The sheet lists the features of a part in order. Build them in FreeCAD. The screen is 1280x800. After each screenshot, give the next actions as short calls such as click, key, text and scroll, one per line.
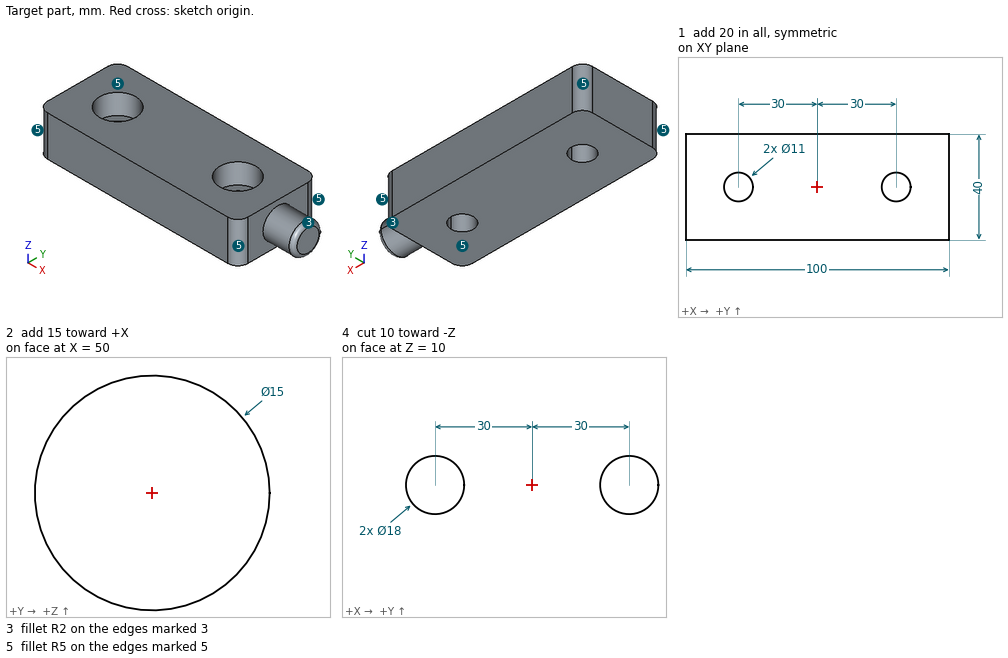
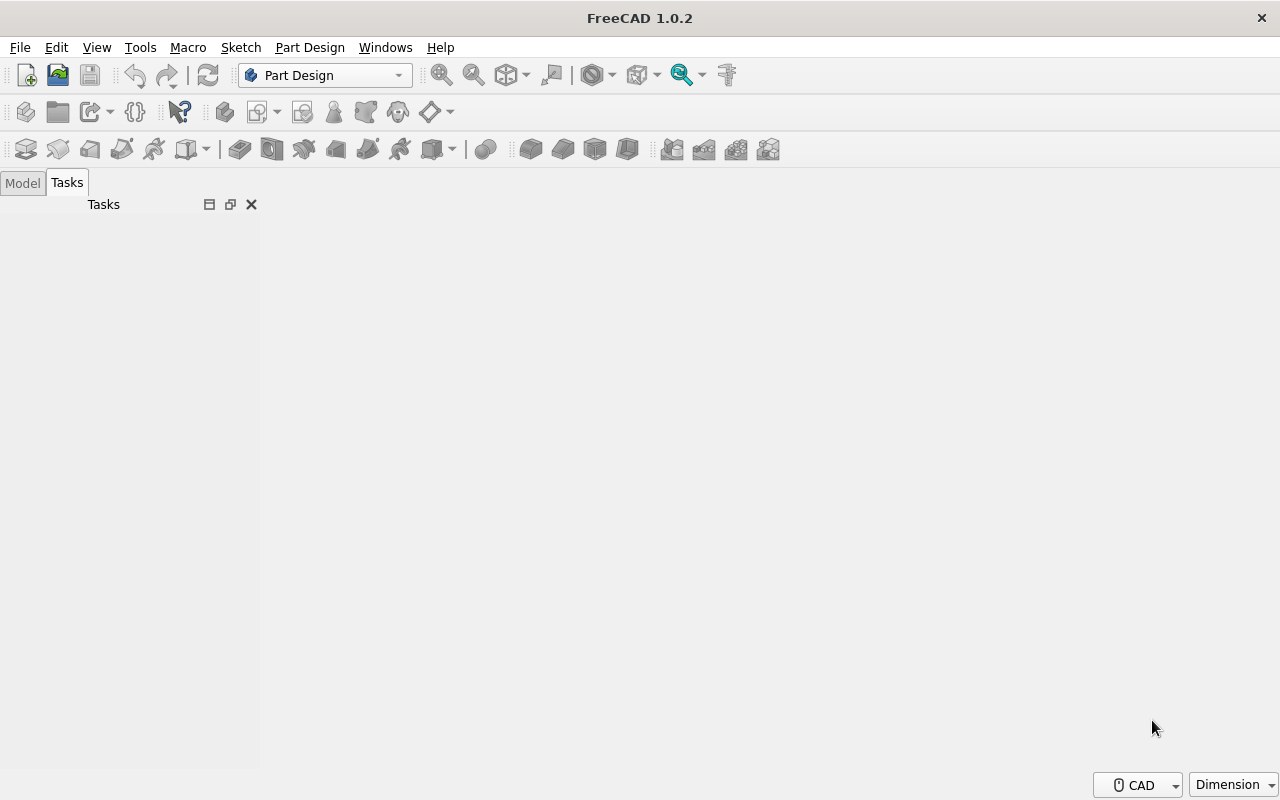
key(ctrl+n)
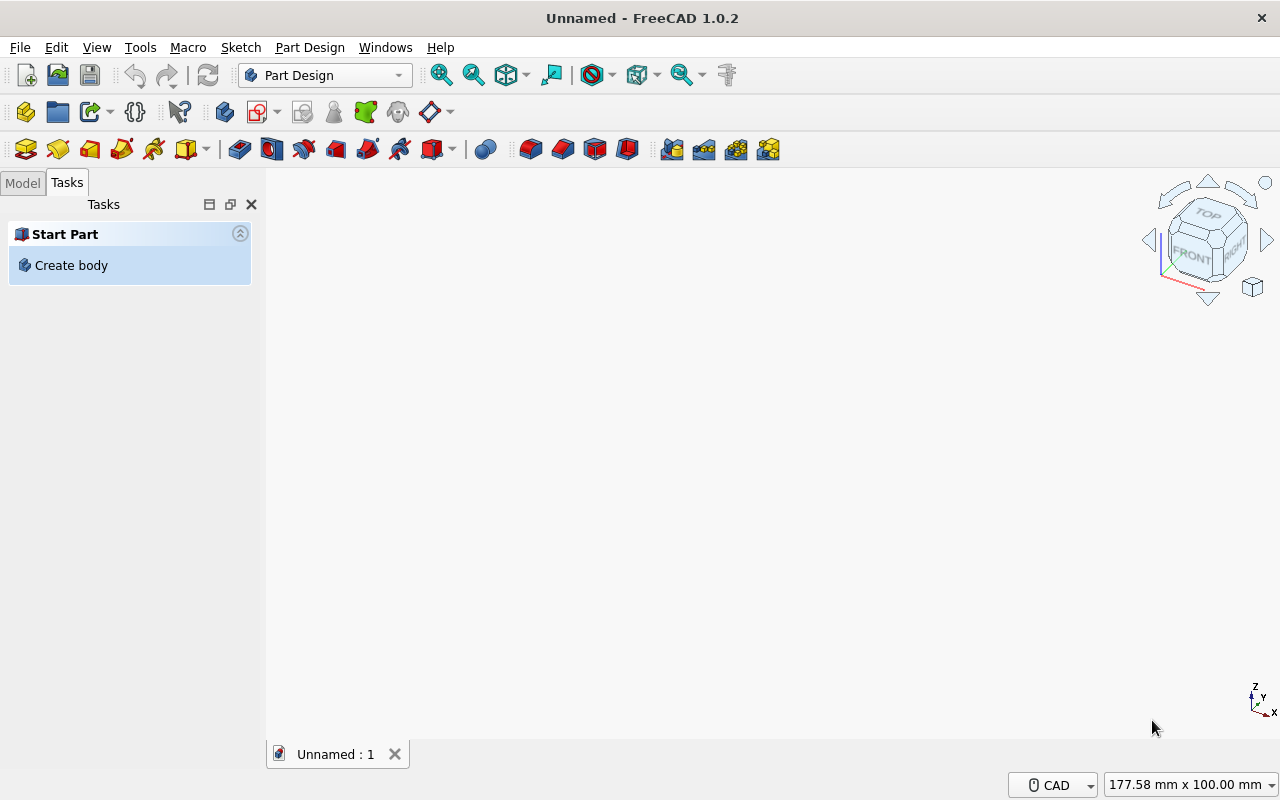
click(258, 112)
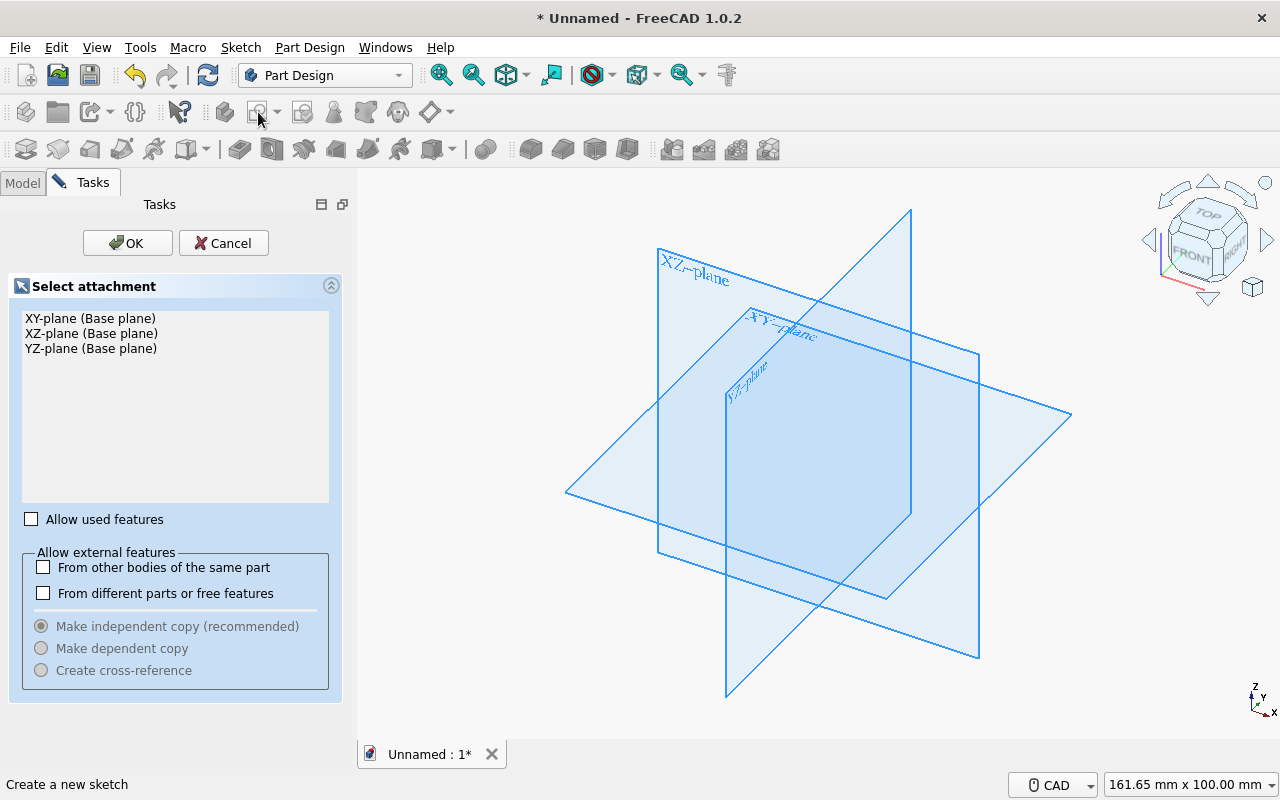
click(82, 318)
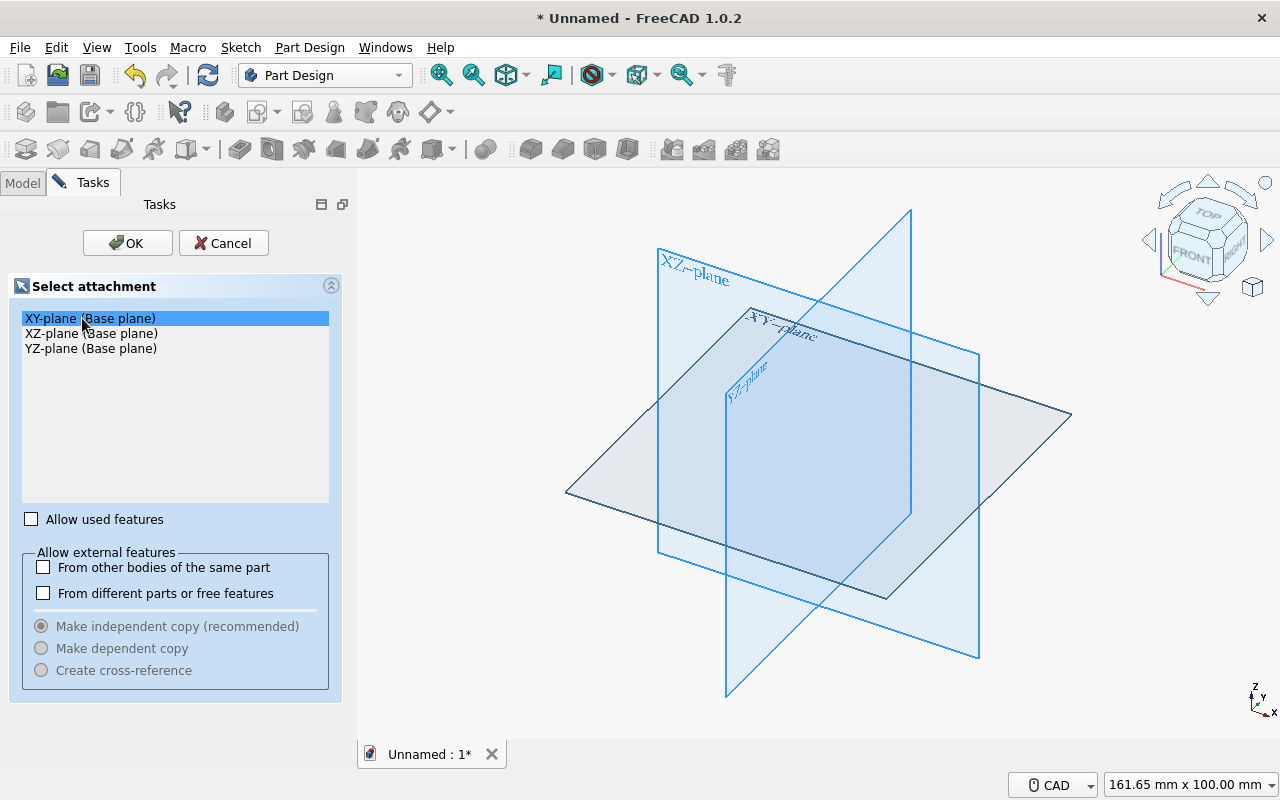
click(128, 243)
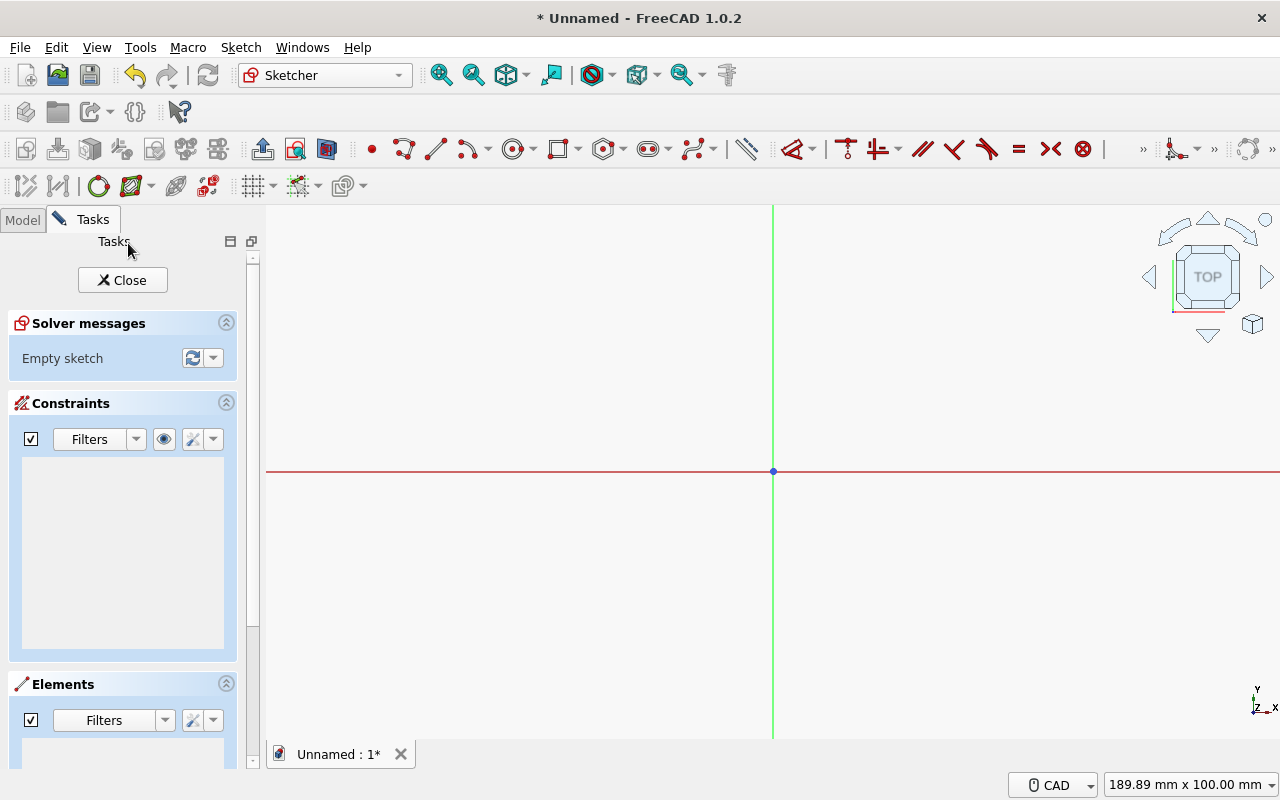
key(g)
key(v)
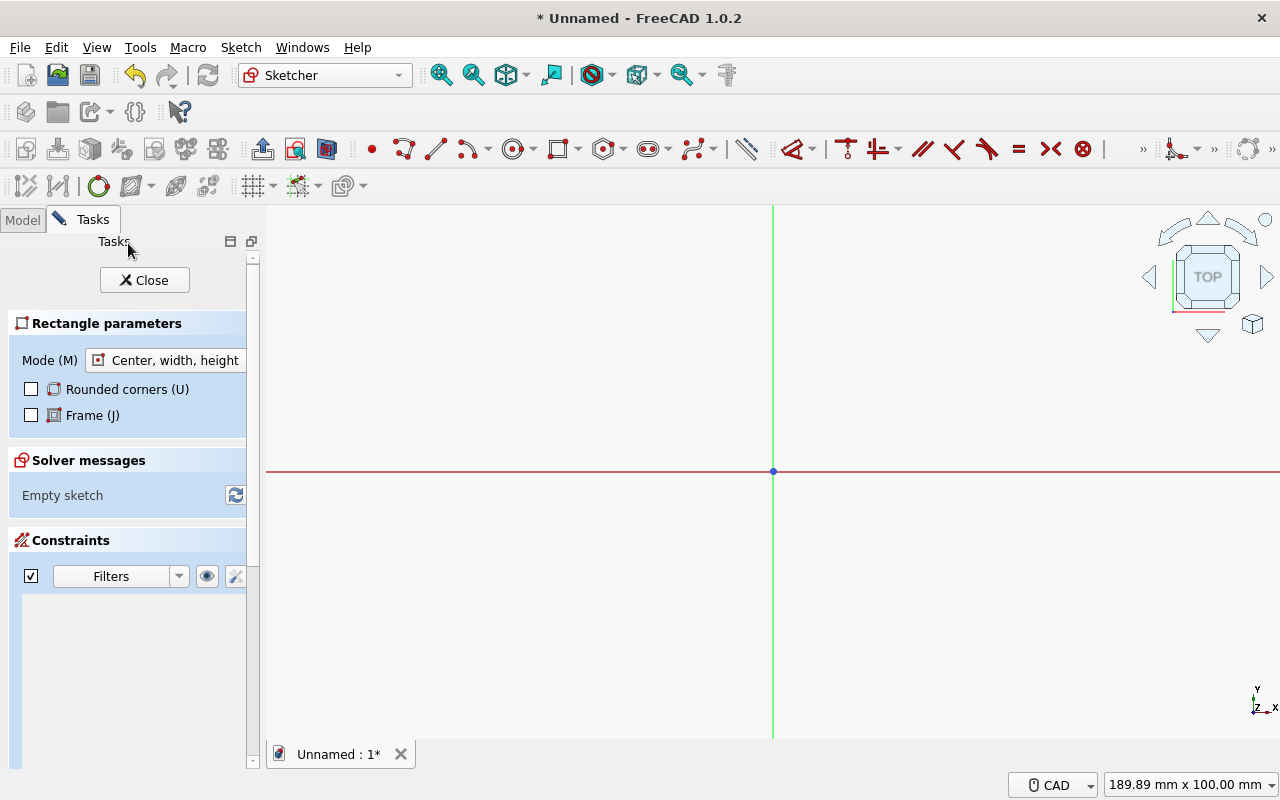
click(773, 472)
click(1040, 365)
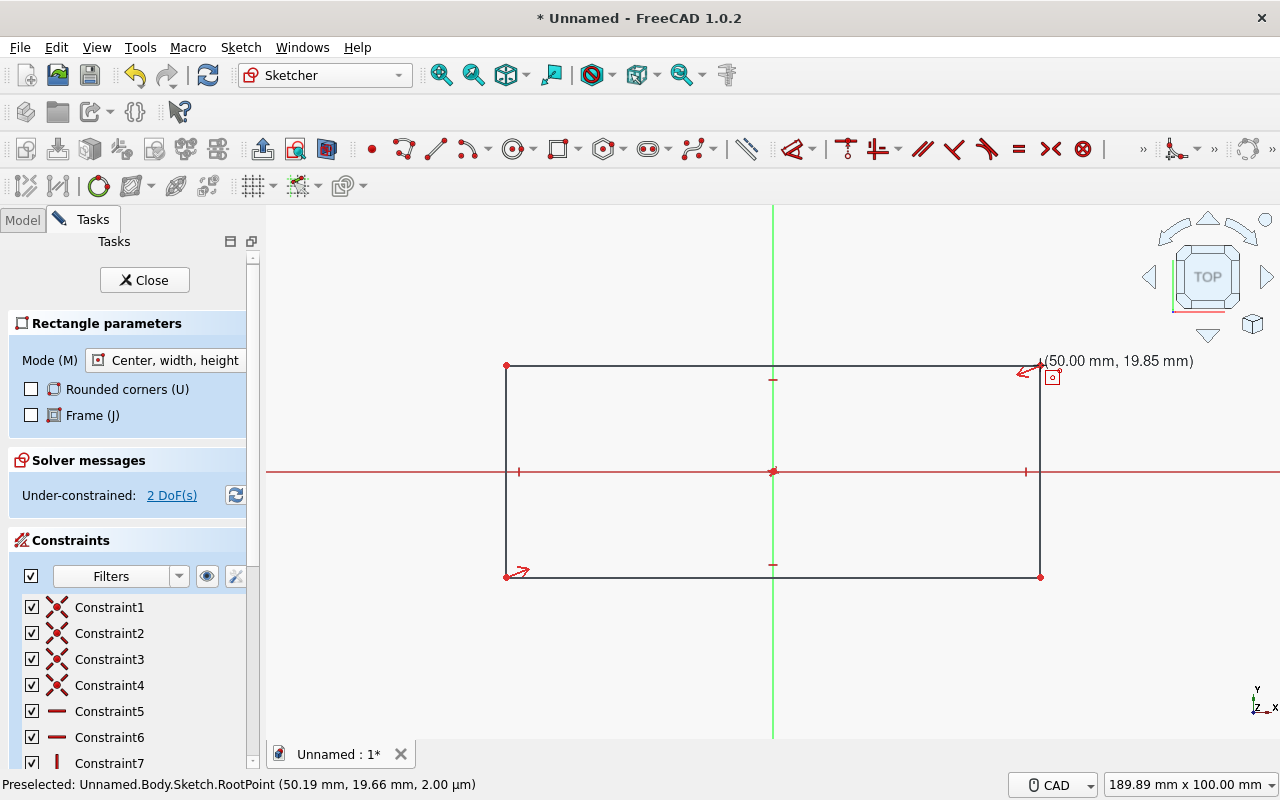
key(g)
key(c)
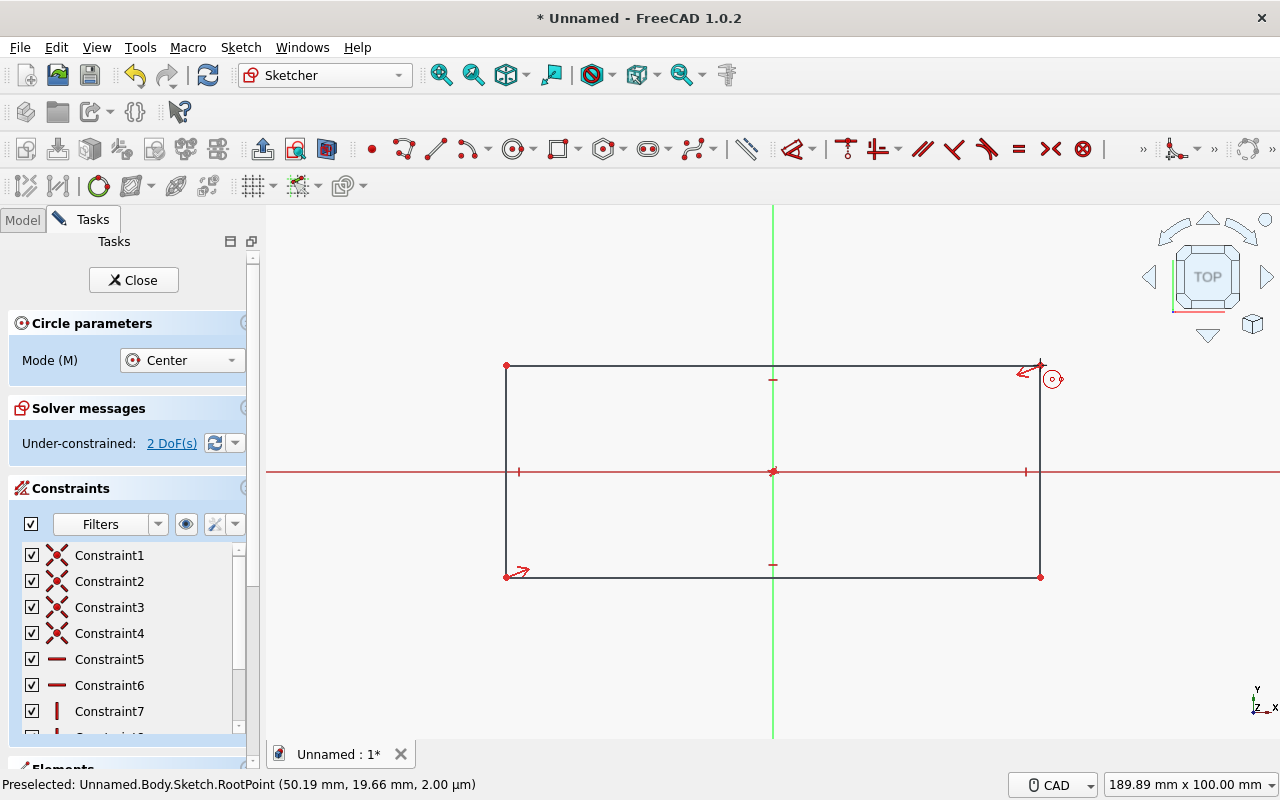
click(613, 472)
click(634, 451)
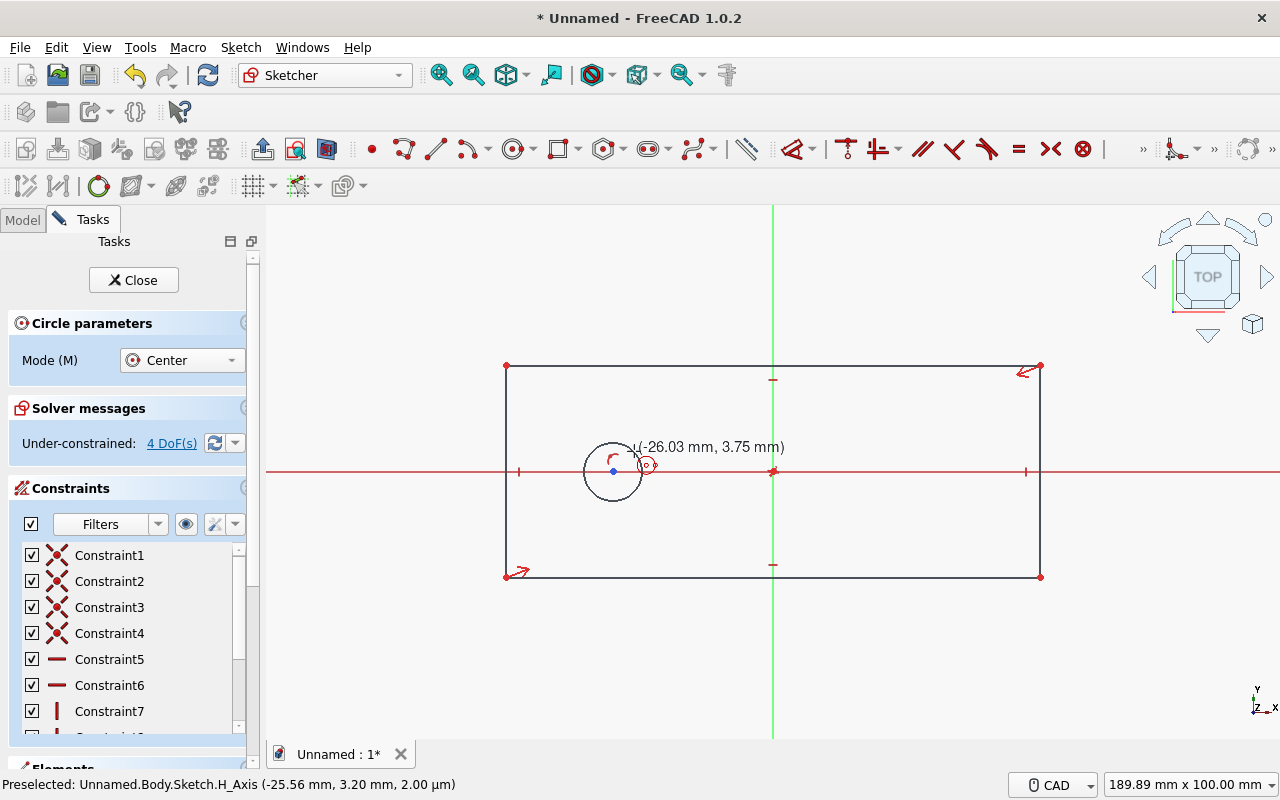
click(933, 472)
click(954, 451)
key(Escape)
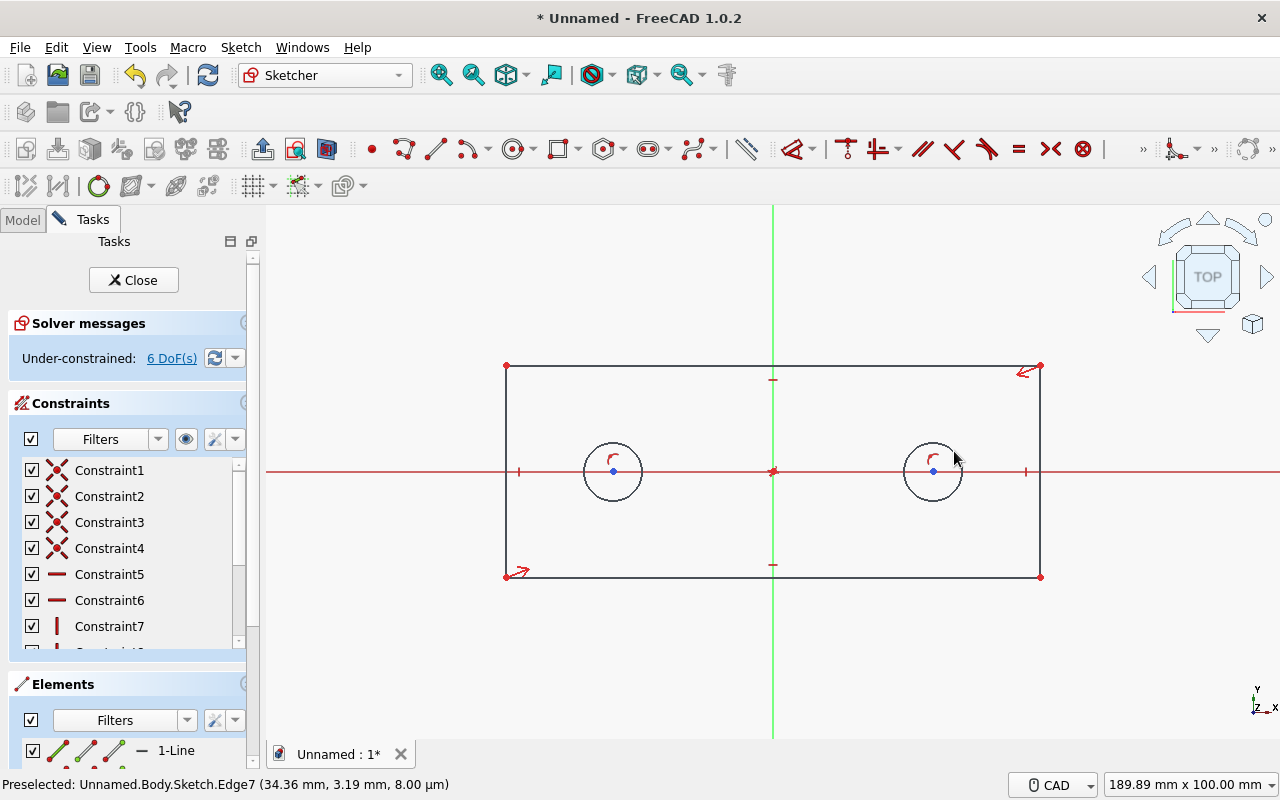
click(633, 451)